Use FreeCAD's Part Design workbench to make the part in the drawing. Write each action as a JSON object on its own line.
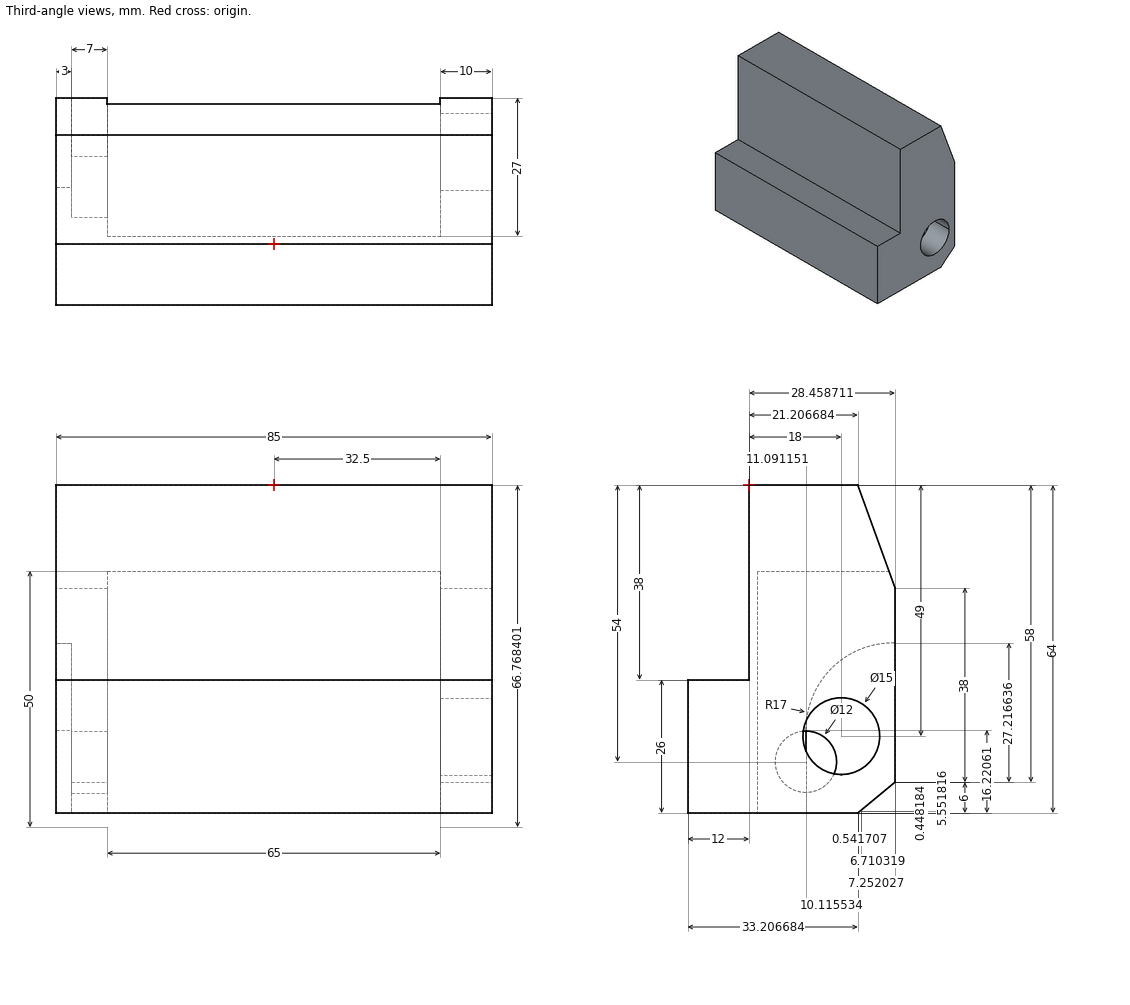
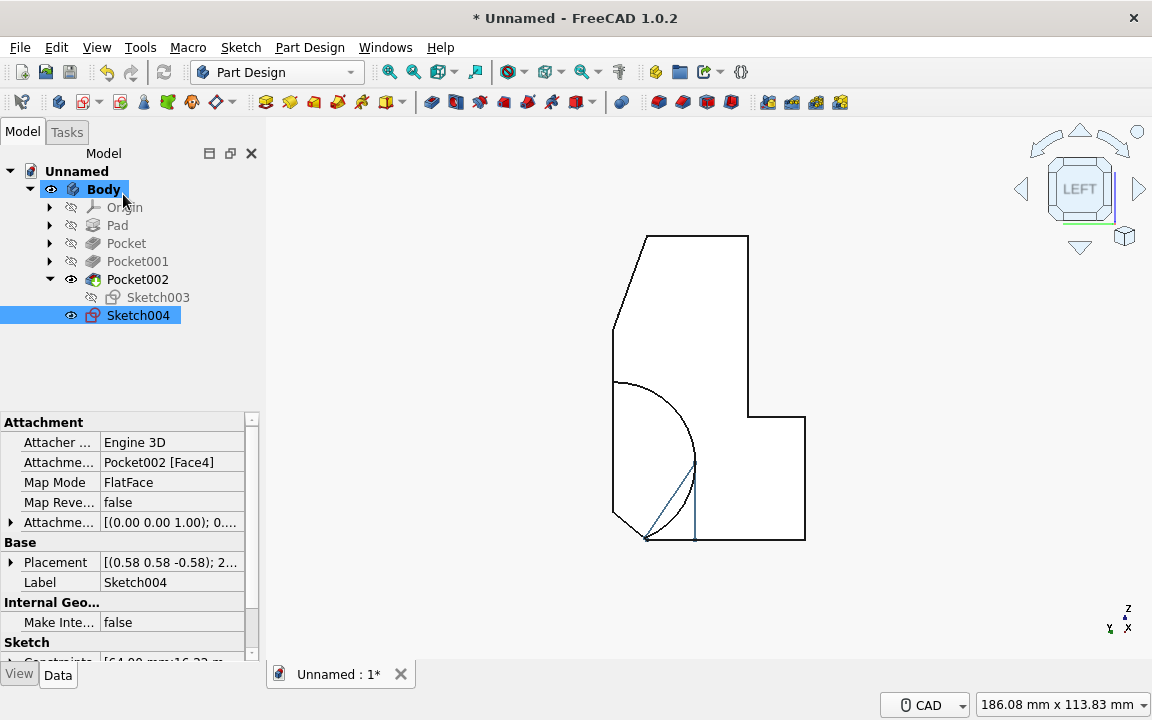
{"action": "left_click", "coordinate": [432, 102]}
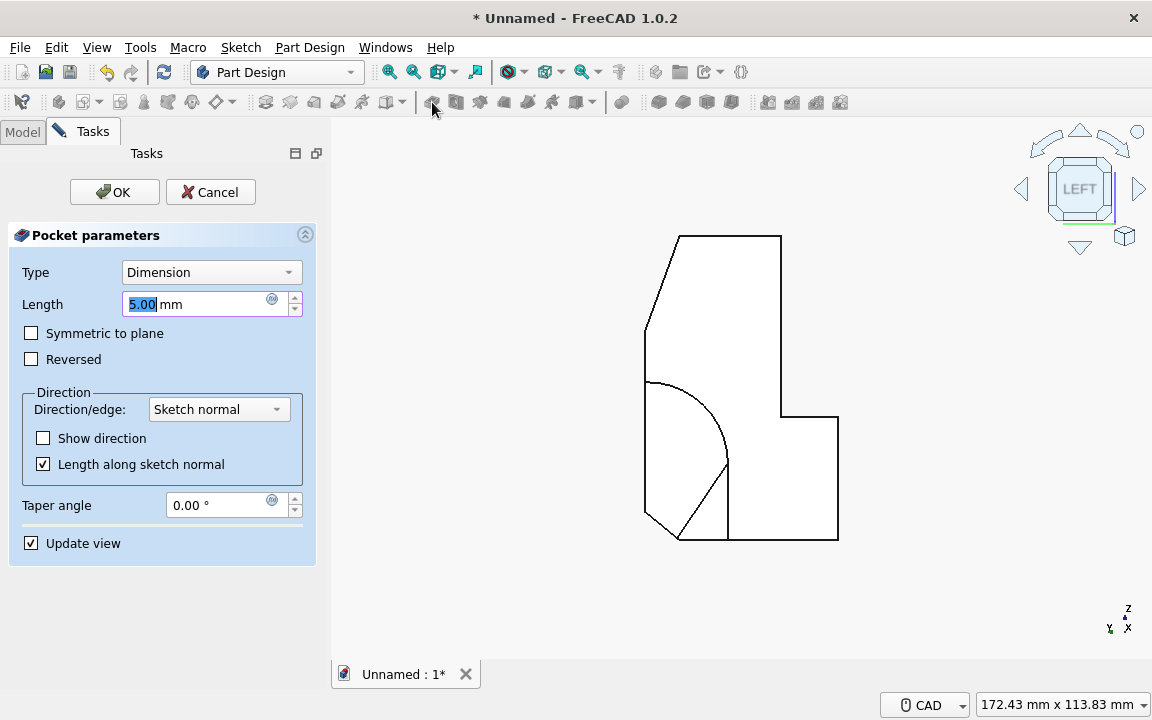
{"action": "type", "text": "3"}
{"action": "key", "text": "Tab"}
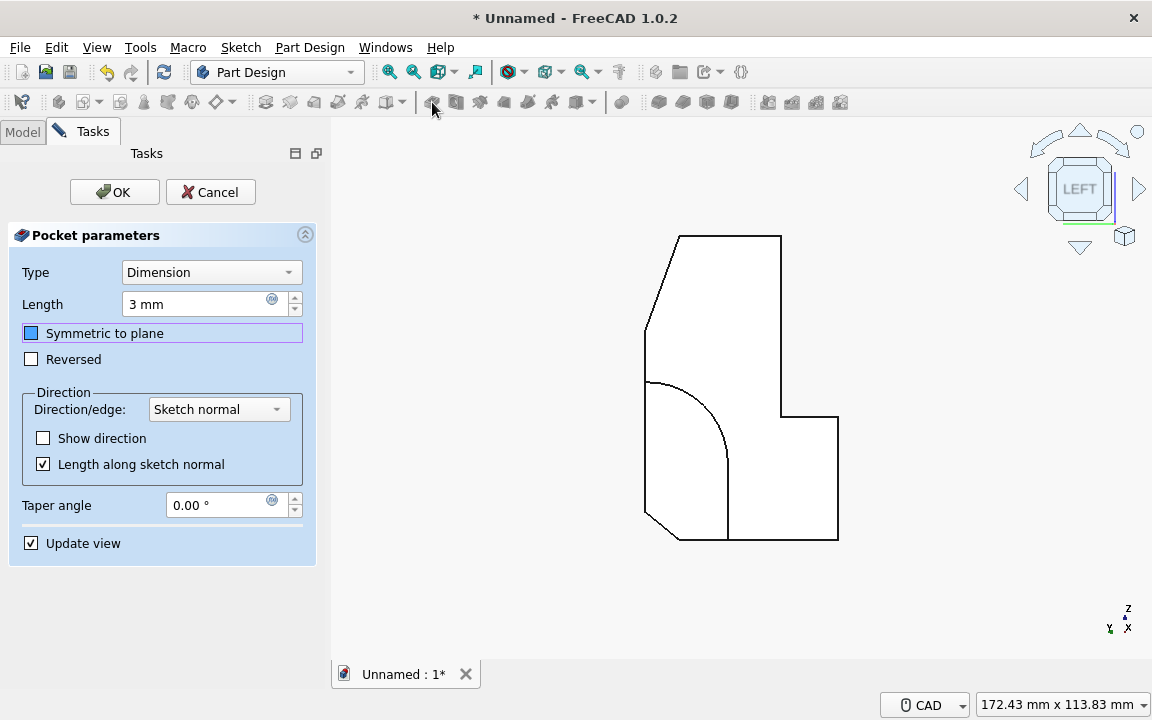
{"action": "left_click", "coordinate": [115, 192]}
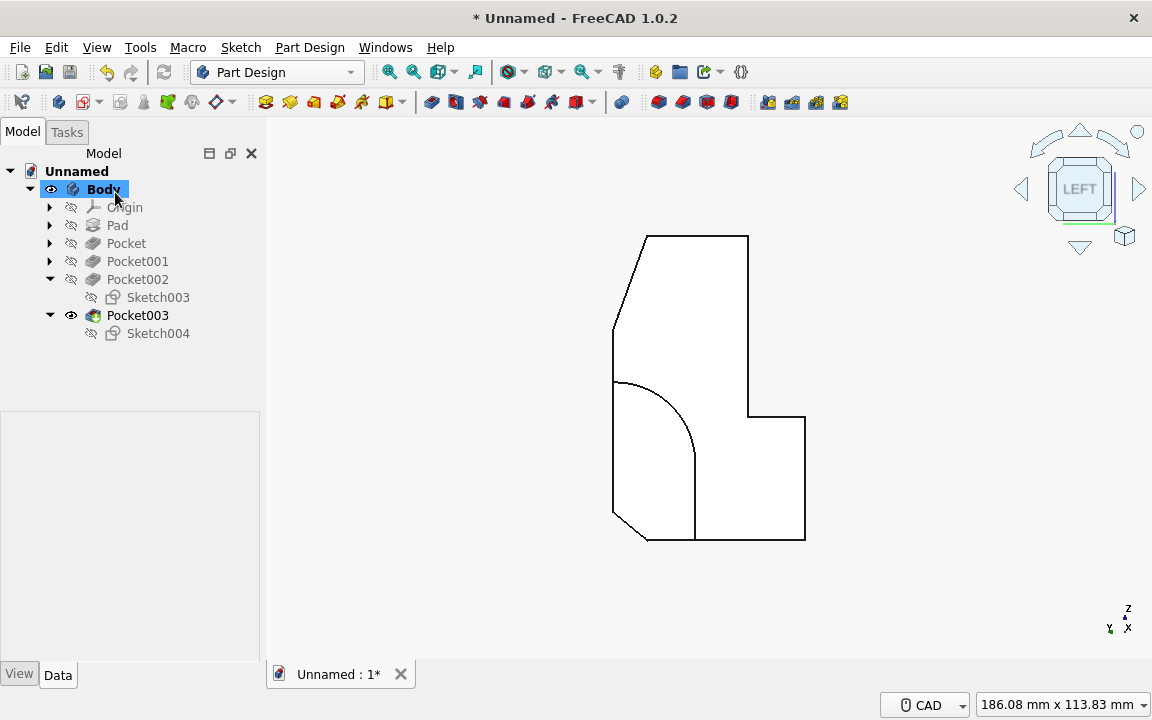
{"action": "left_click", "coordinate": [654, 483]}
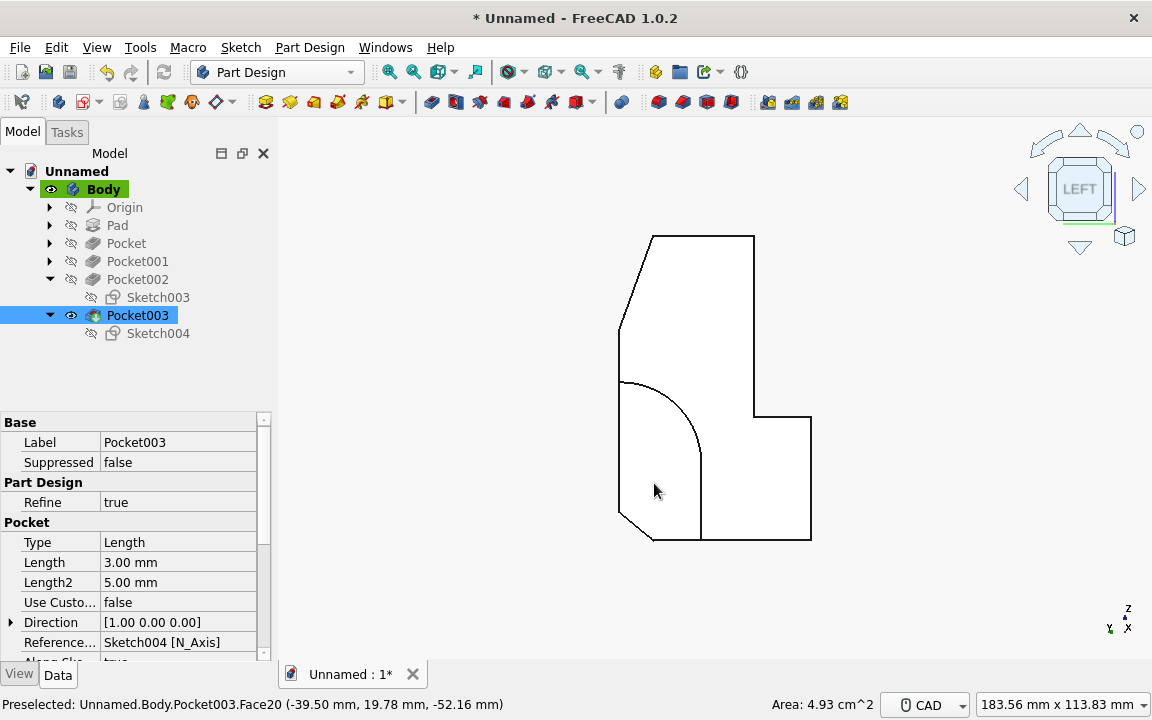
{"action": "left_click", "coordinate": [84, 102]}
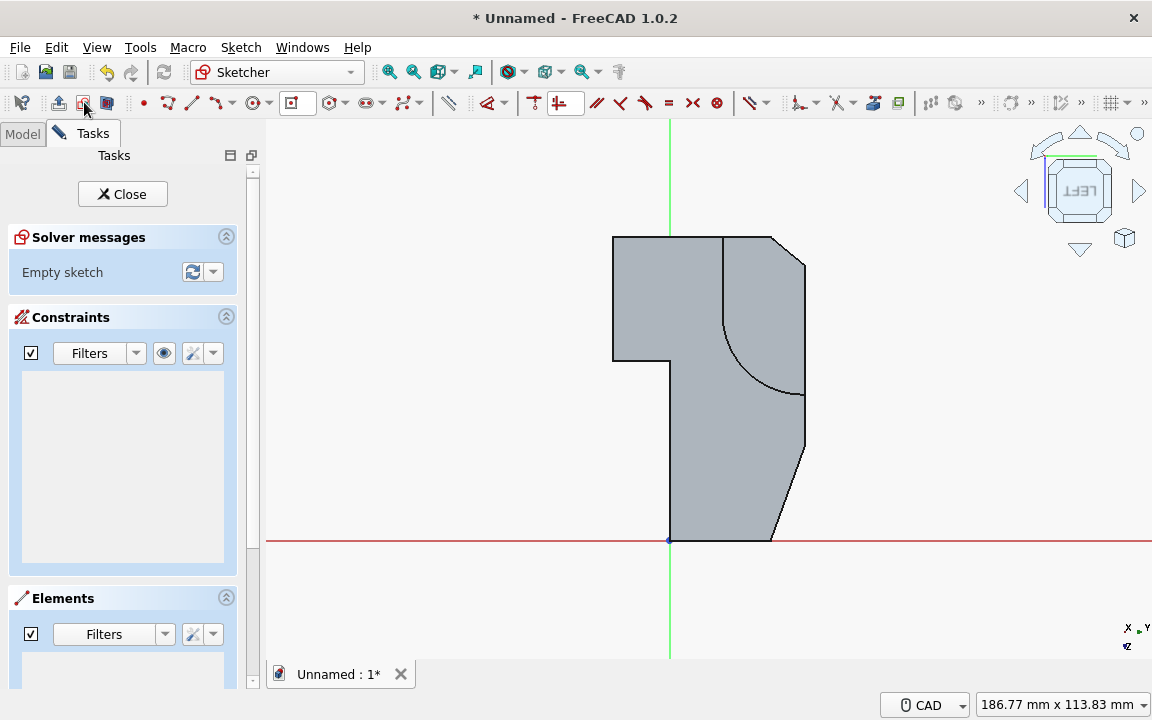
{"action": "scroll", "coordinate": [739, 264], "scroll_direction": "up", "scroll_amount": 9}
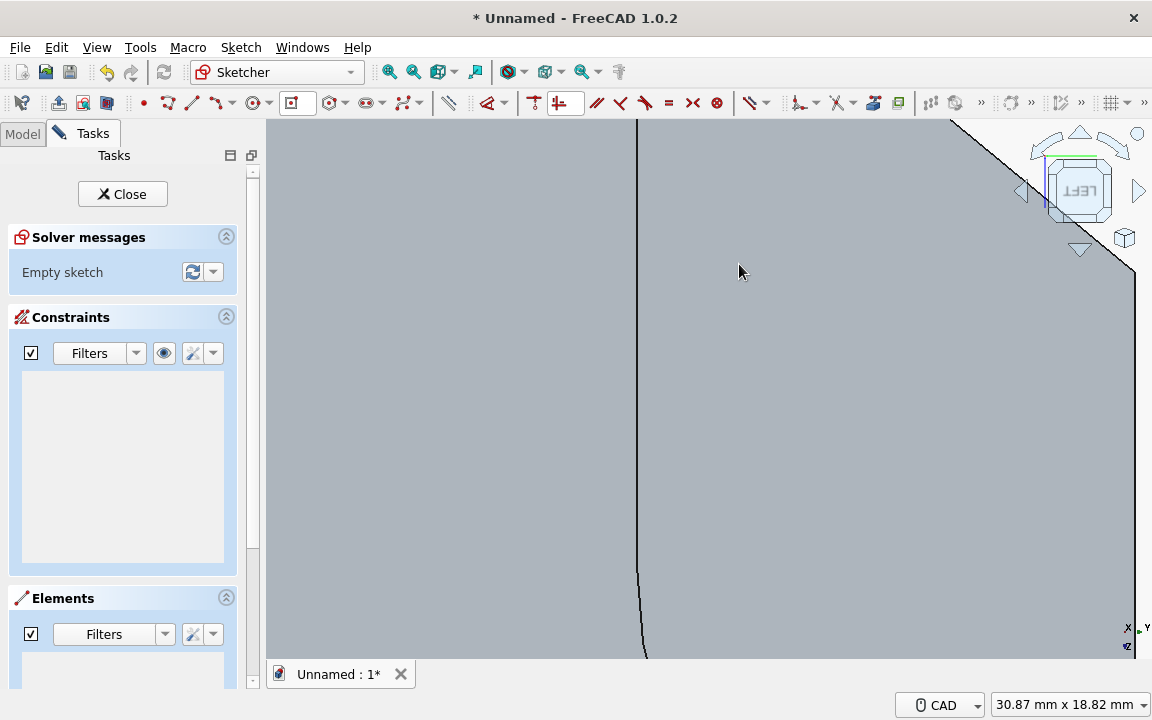
{"action": "left_click", "coordinate": [254, 104]}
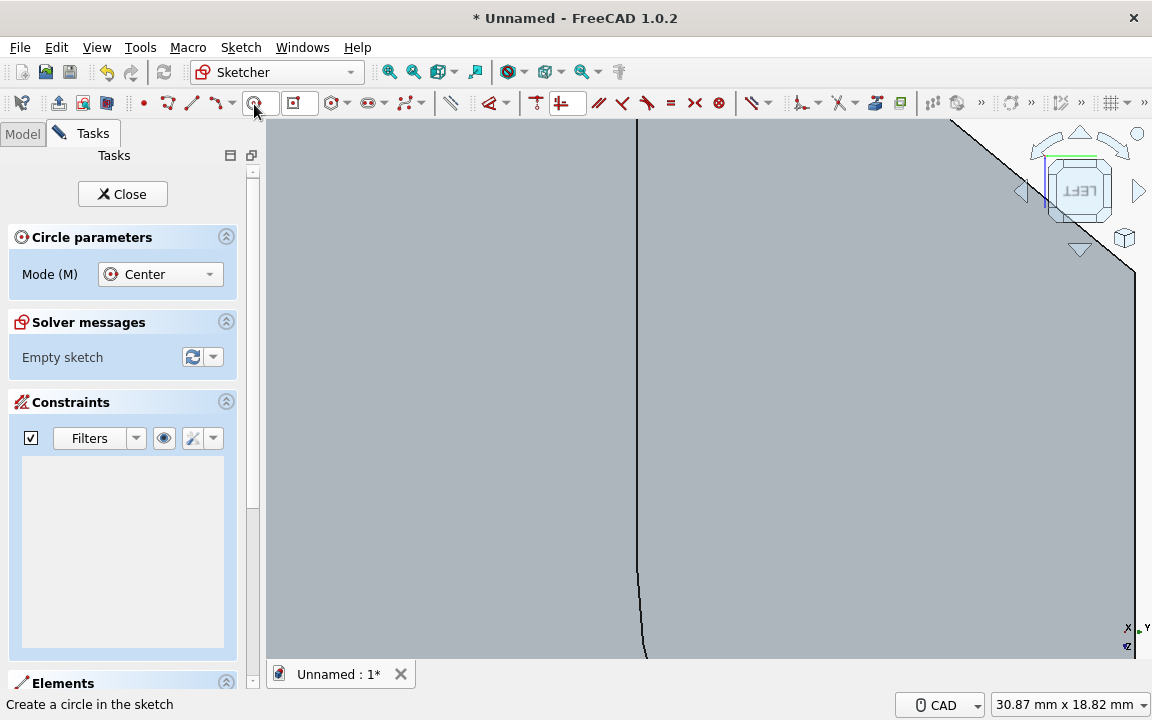
{"action": "left_click", "coordinate": [637, 387]}
{"action": "left_click", "coordinate": [759, 266]}
{"action": "key", "text": "Escape"}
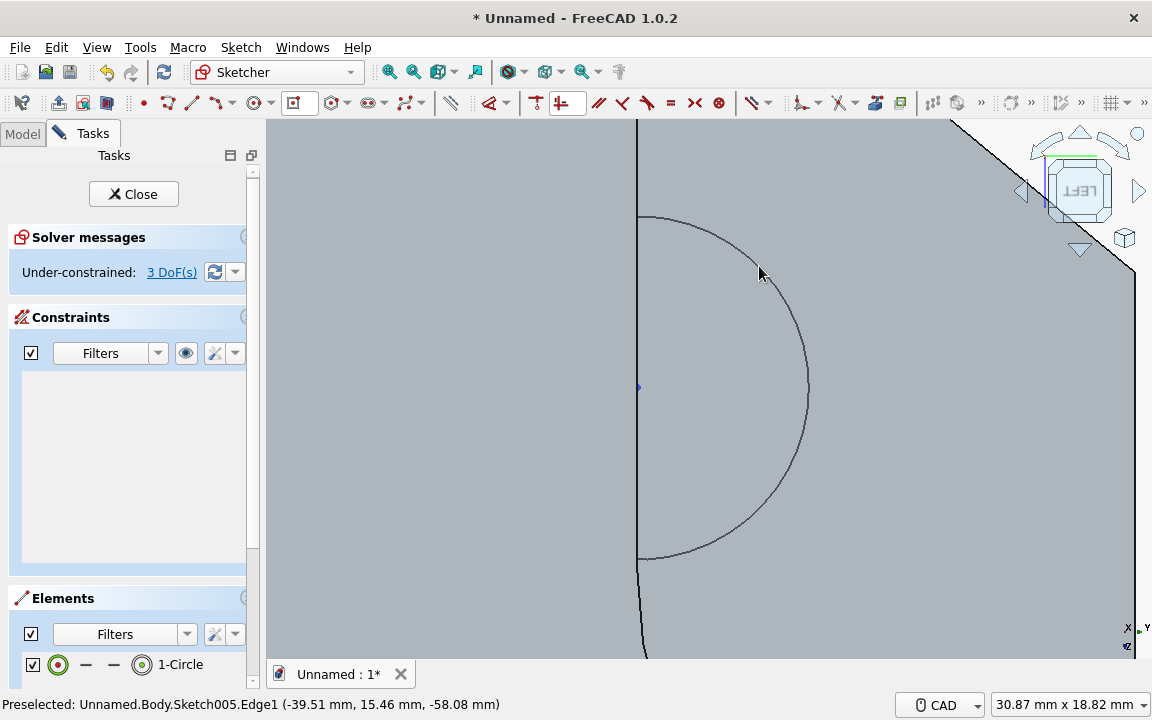
{"action": "left_click", "coordinate": [490, 104]}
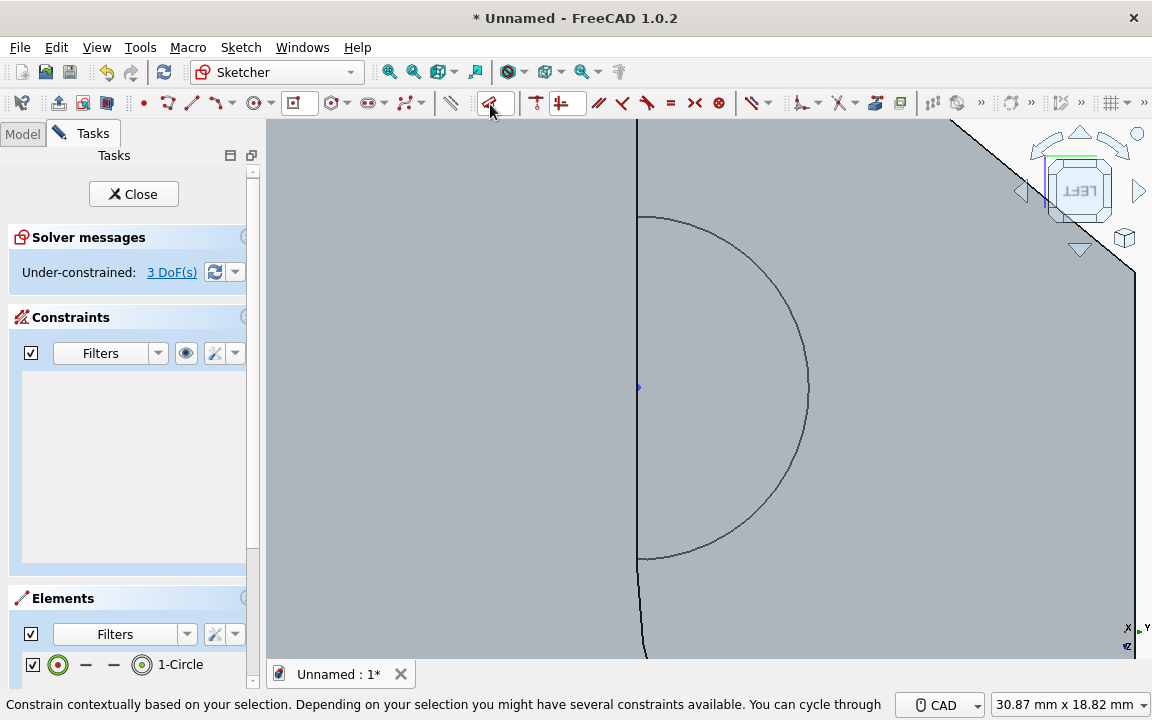
{"action": "left_click", "coordinate": [758, 266]}
{"action": "left_click", "coordinate": [781, 243]}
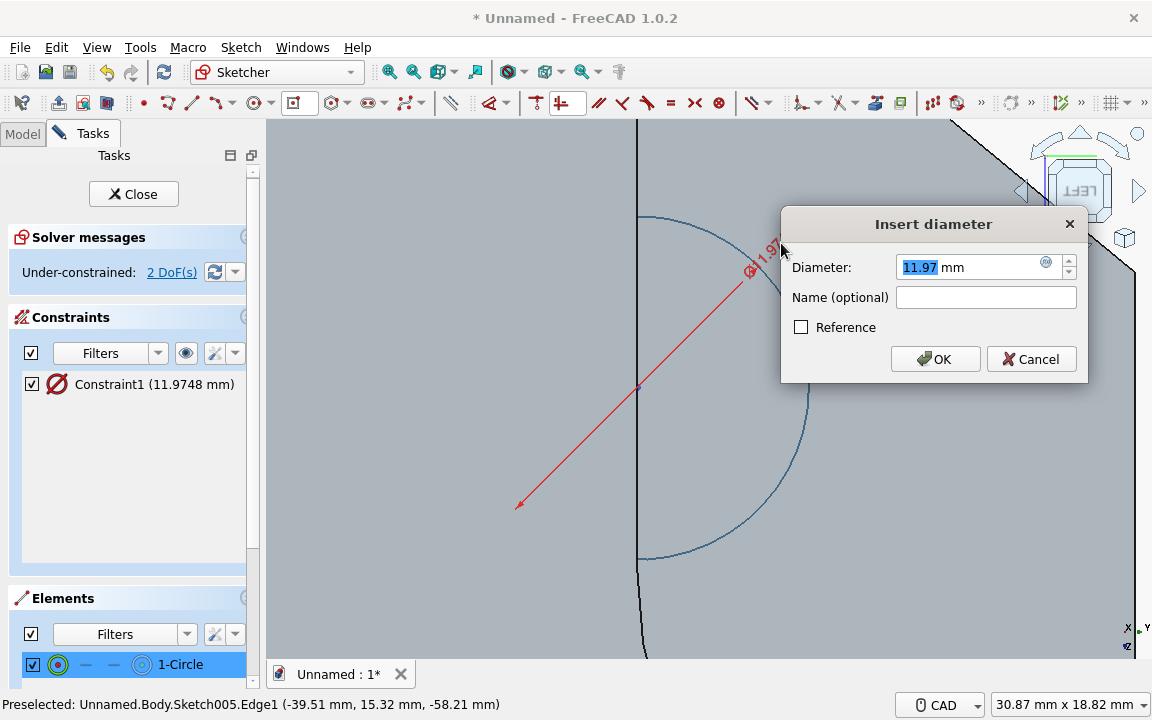
{"action": "type", "text": "12"}
{"action": "key", "text": "Return"}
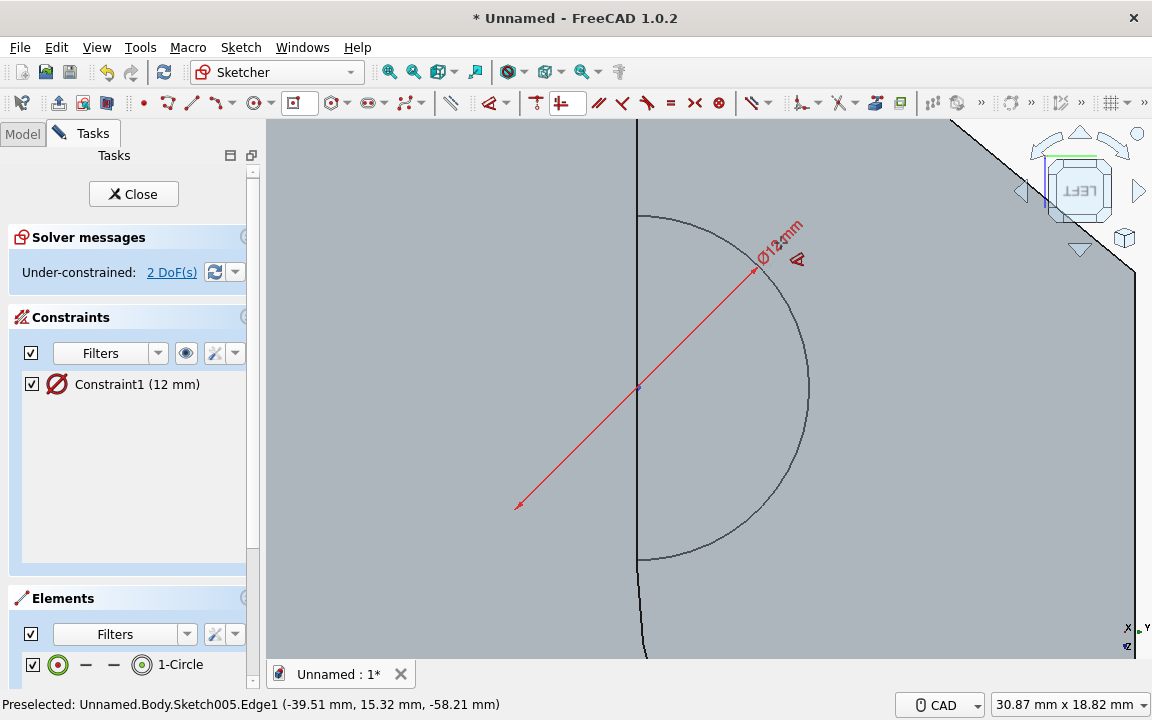
{"action": "left_click", "coordinate": [637, 388]}
{"action": "left_click", "coordinate": [671, 510]}